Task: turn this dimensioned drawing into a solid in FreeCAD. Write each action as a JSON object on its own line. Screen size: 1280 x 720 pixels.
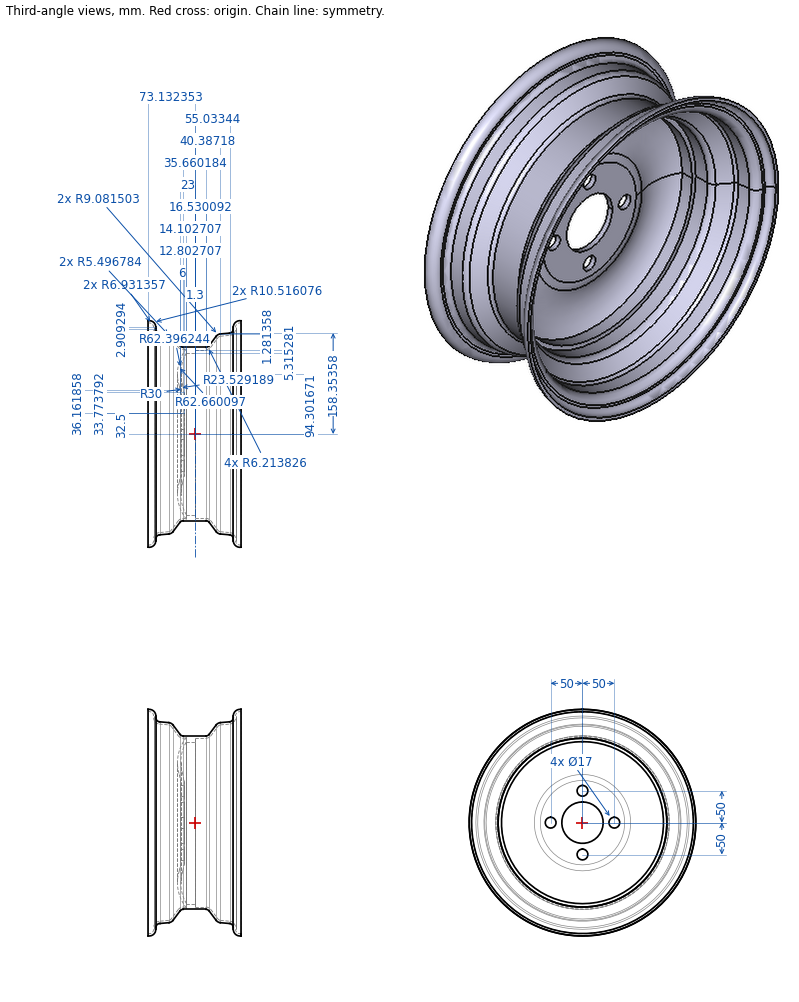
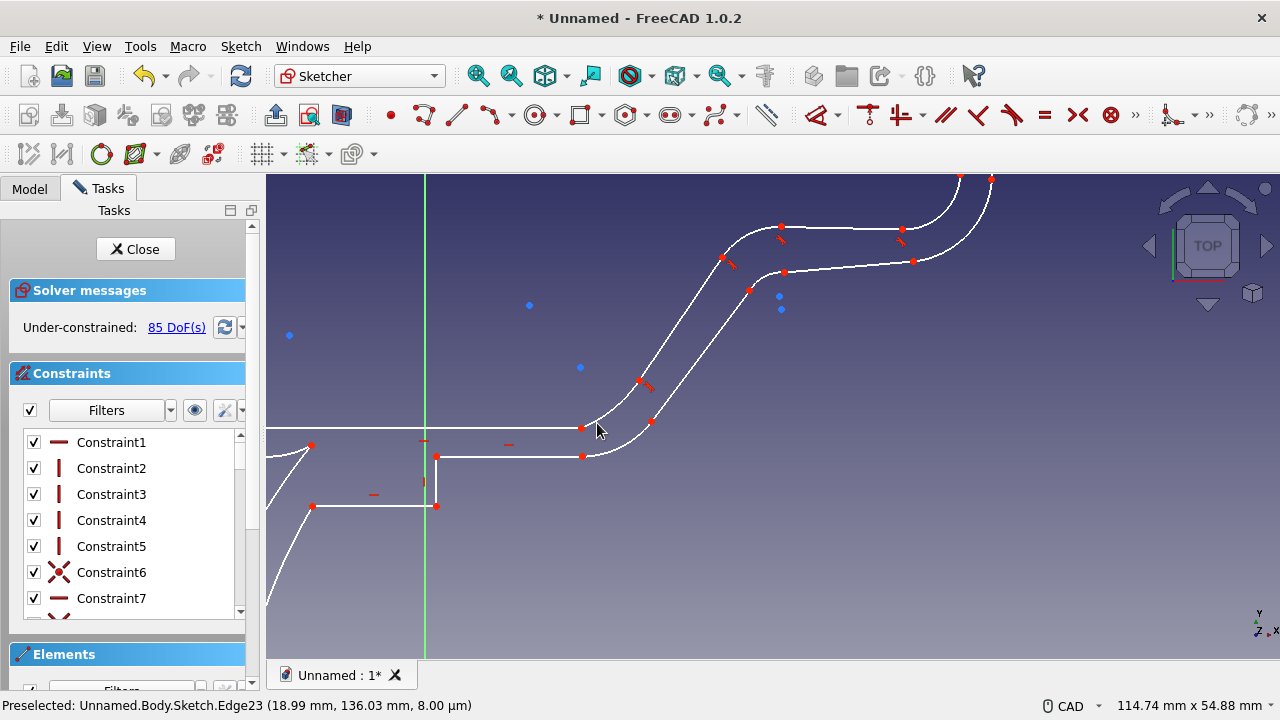
{"action": "left_click", "coordinate": [487, 428]}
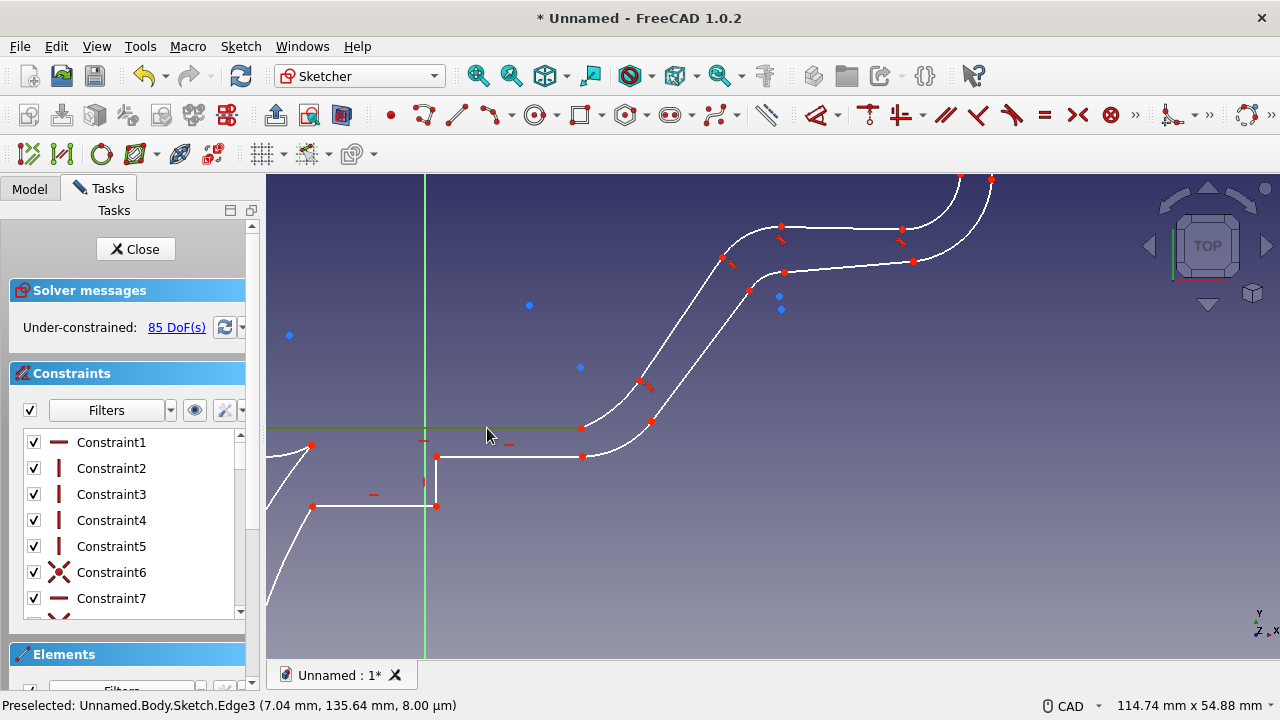
{"action": "left_click", "coordinate": [602, 417]}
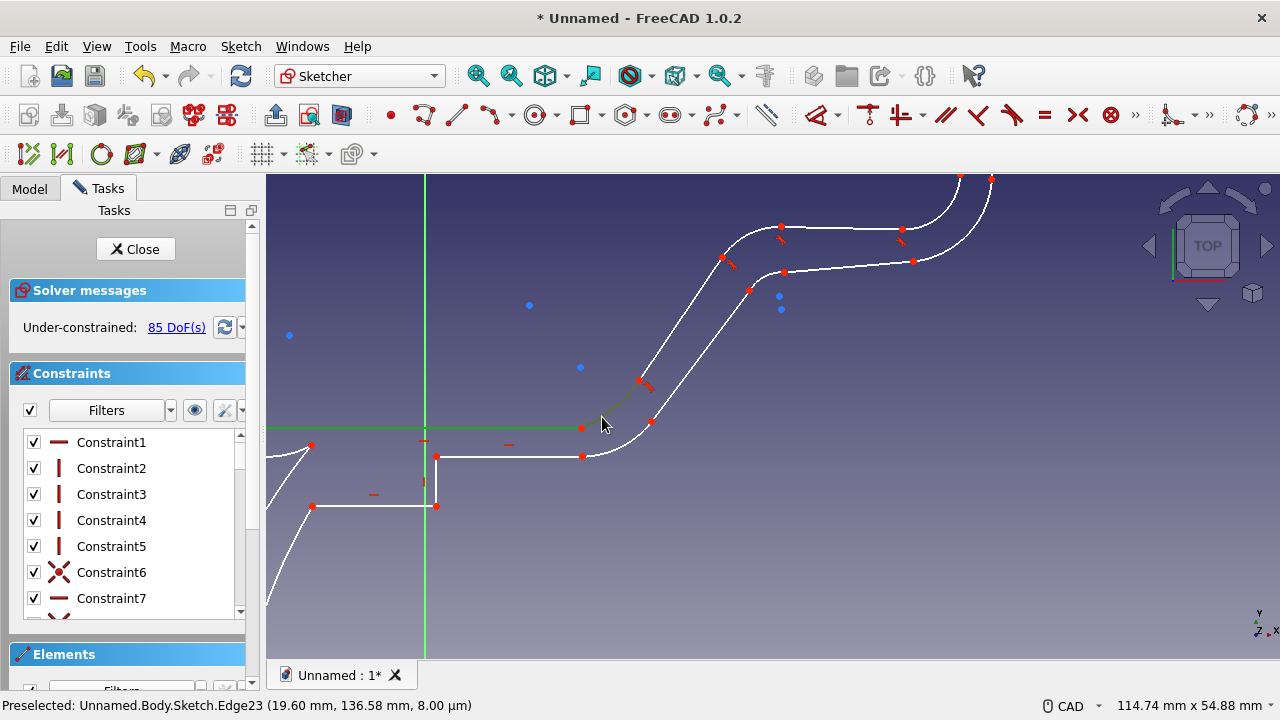
{"action": "key", "text": "t"}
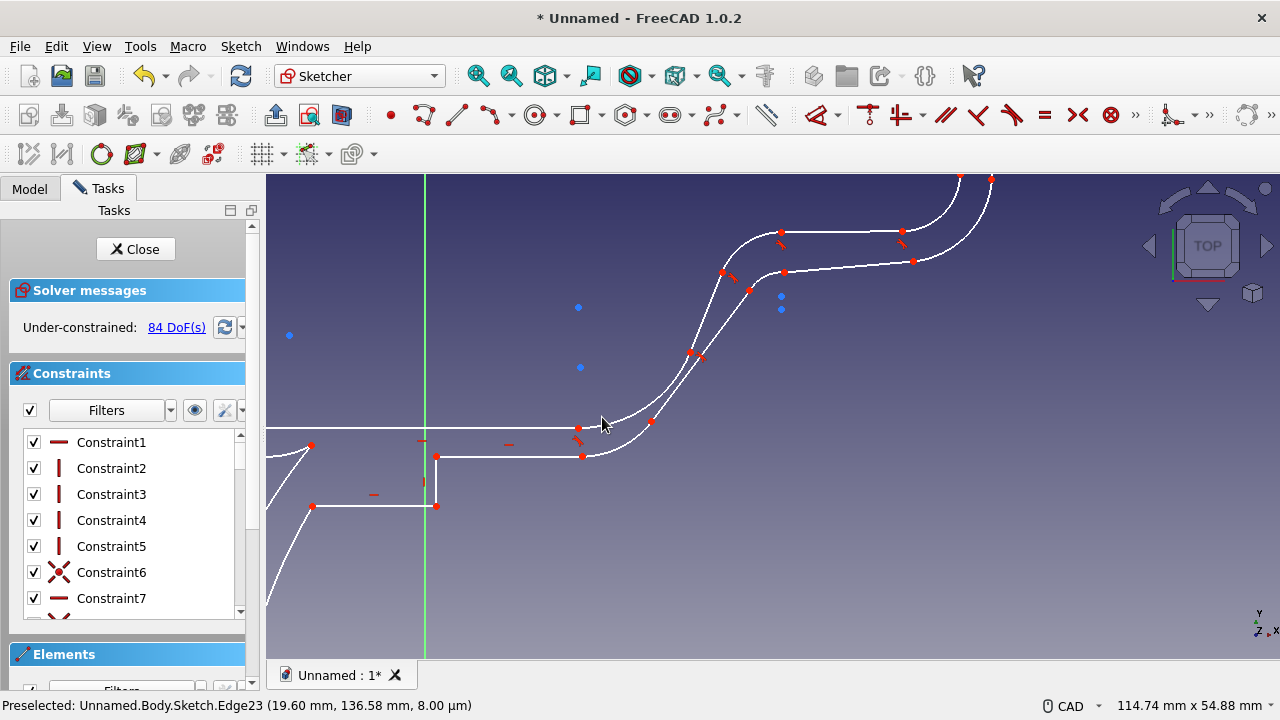
{"action": "left_click", "coordinate": [485, 428]}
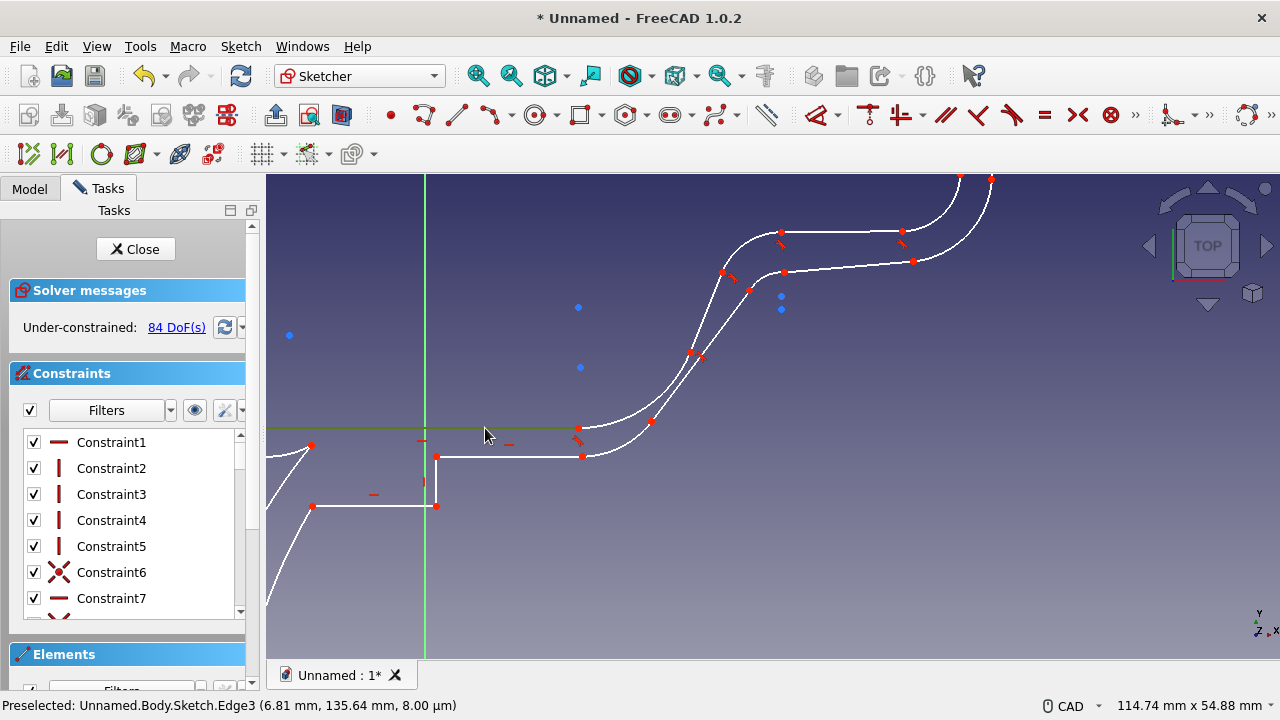
{"action": "scroll", "coordinate": [775, 309], "scroll_direction": "down", "scroll_amount": 8}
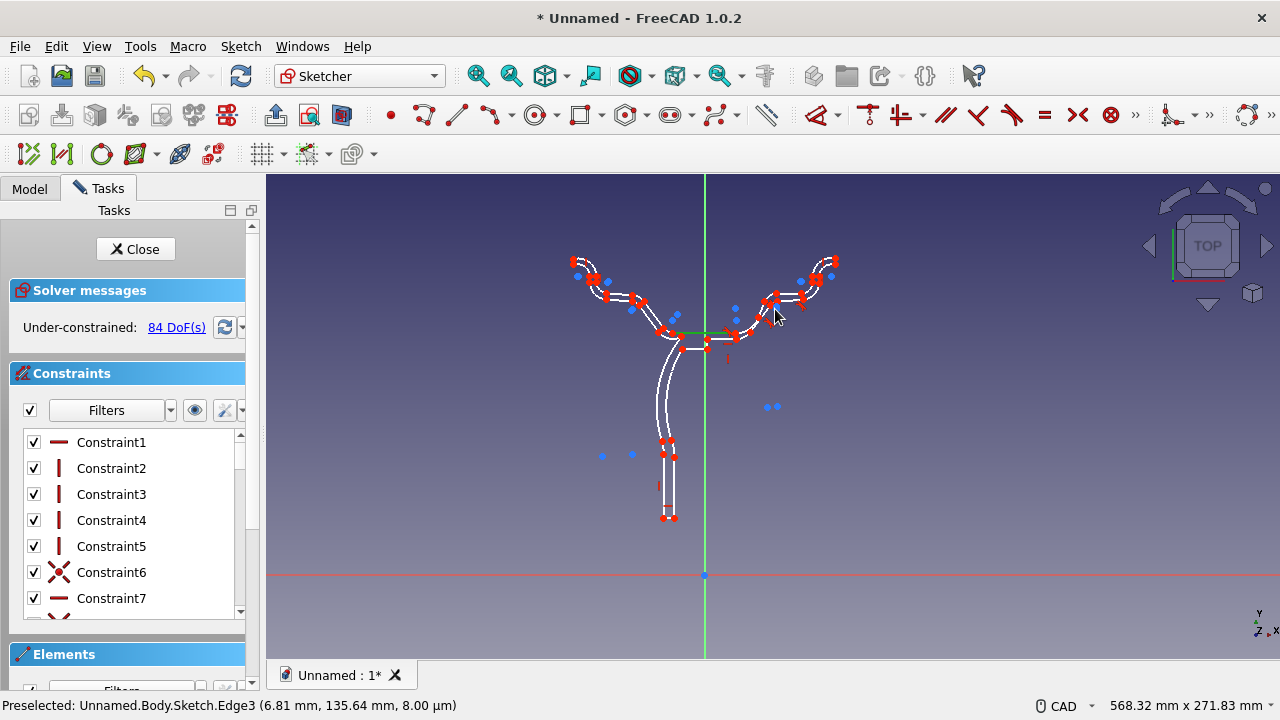
{"action": "scroll", "coordinate": [666, 330], "scroll_direction": "up", "scroll_amount": 8}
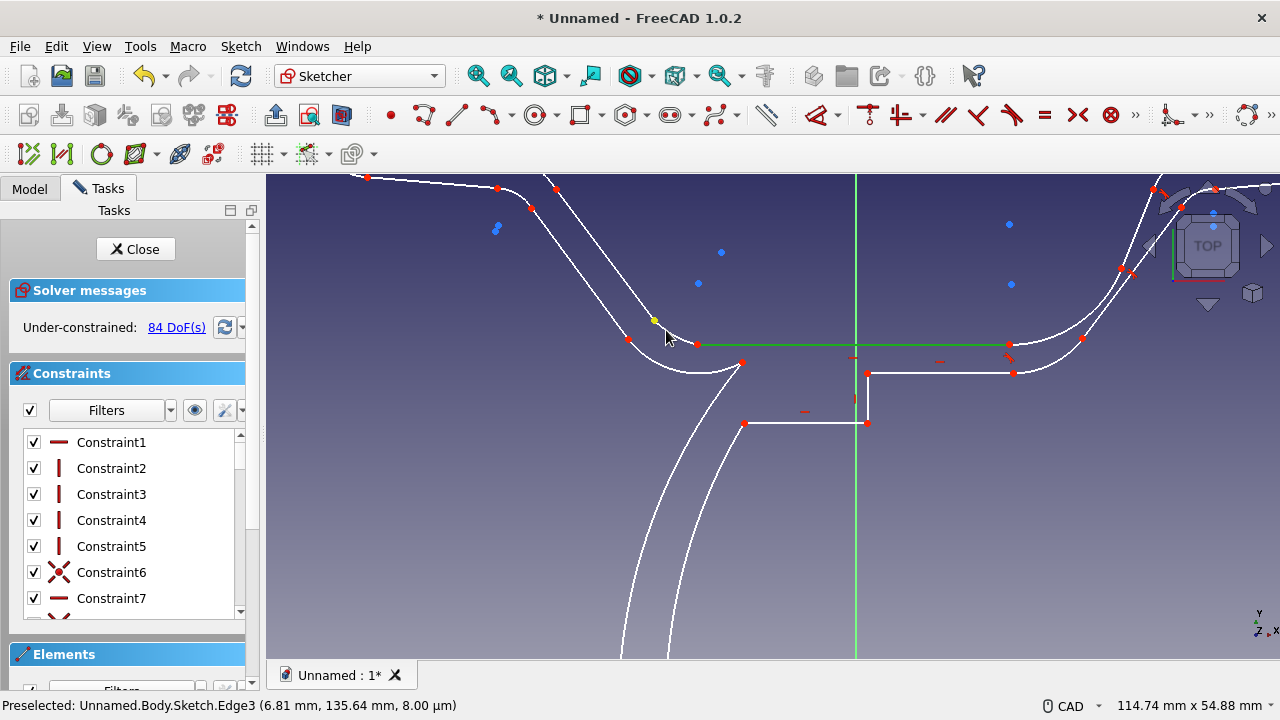
{"action": "left_click", "coordinate": [666, 330]}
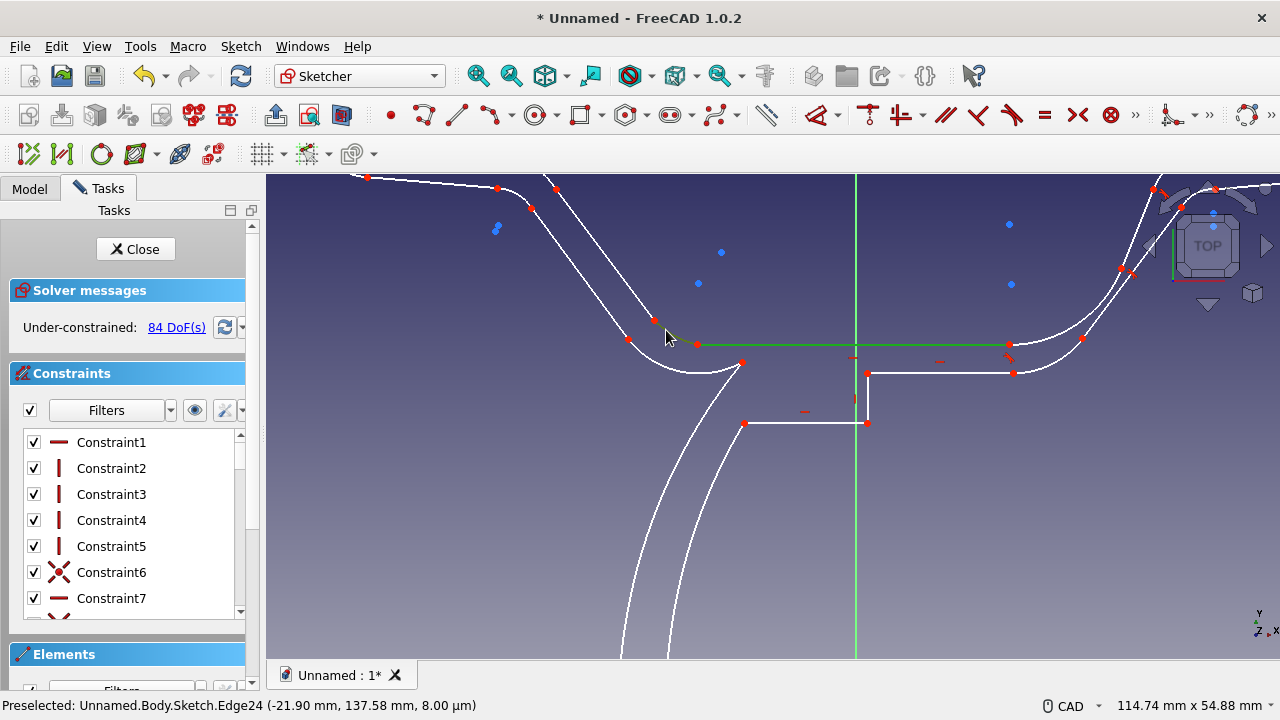
{"action": "key", "text": "t"}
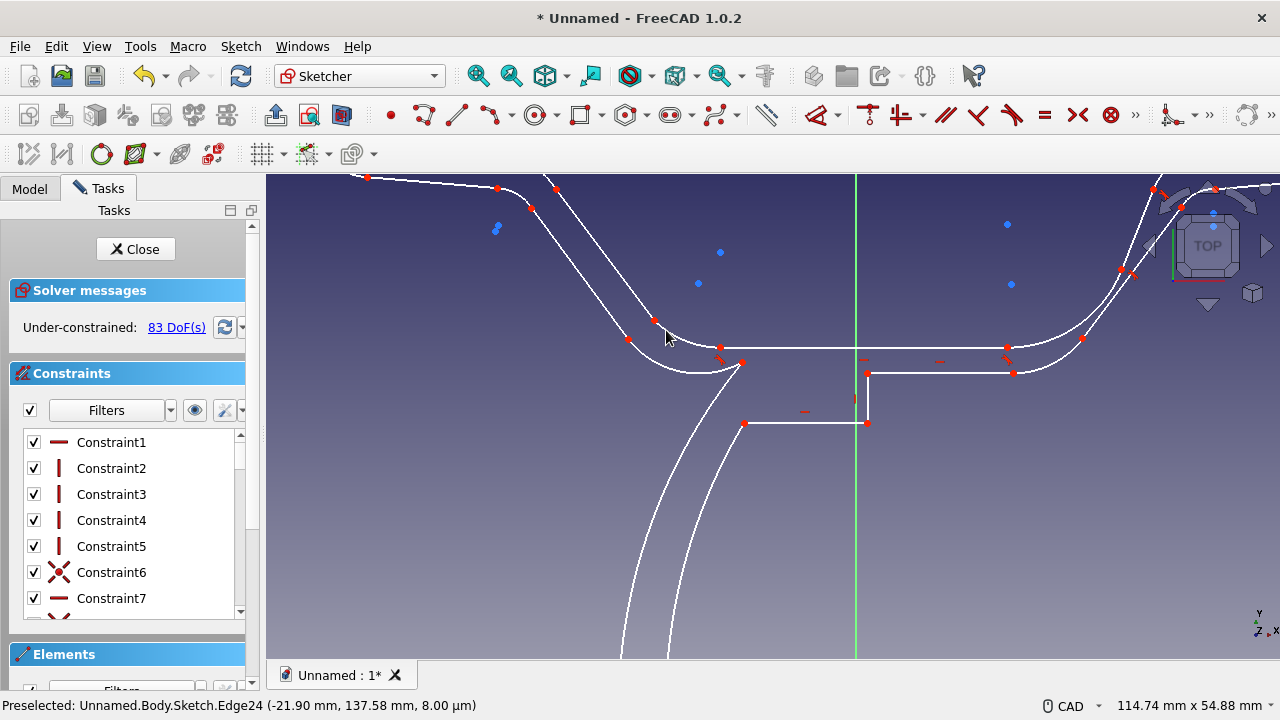
{"action": "left_click", "coordinate": [625, 281]}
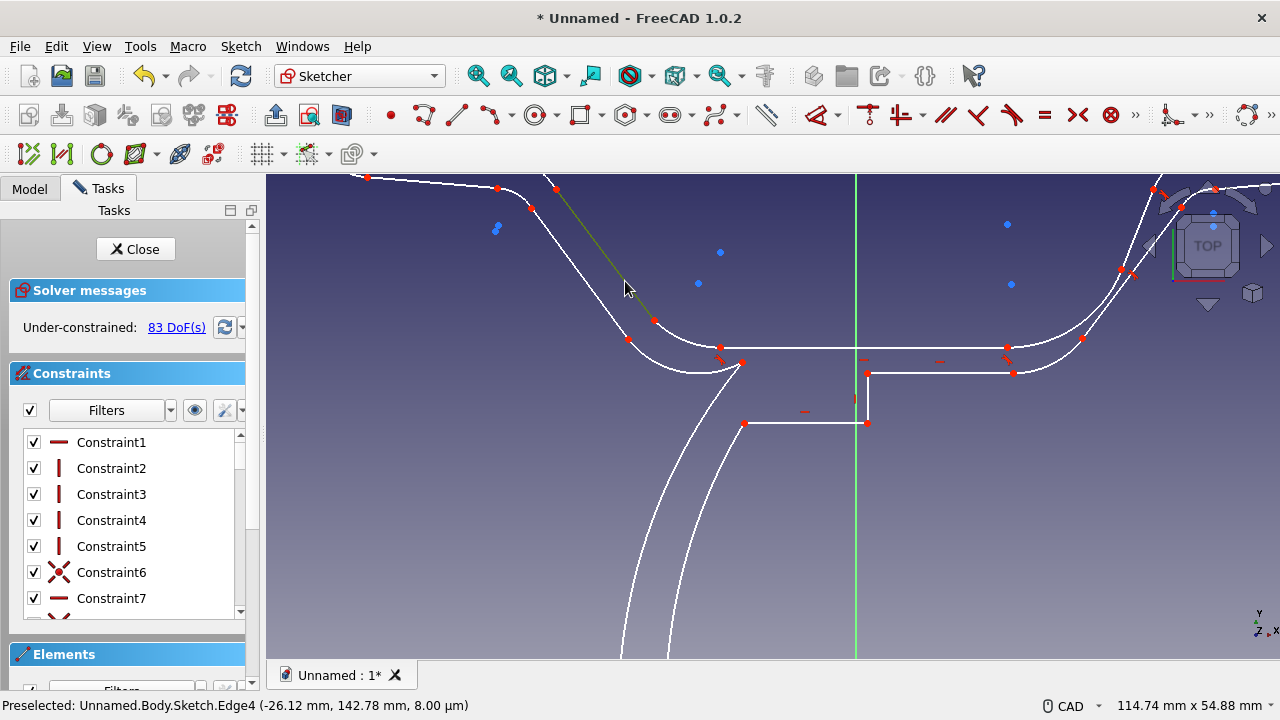
{"action": "left_click", "coordinate": [672, 334]}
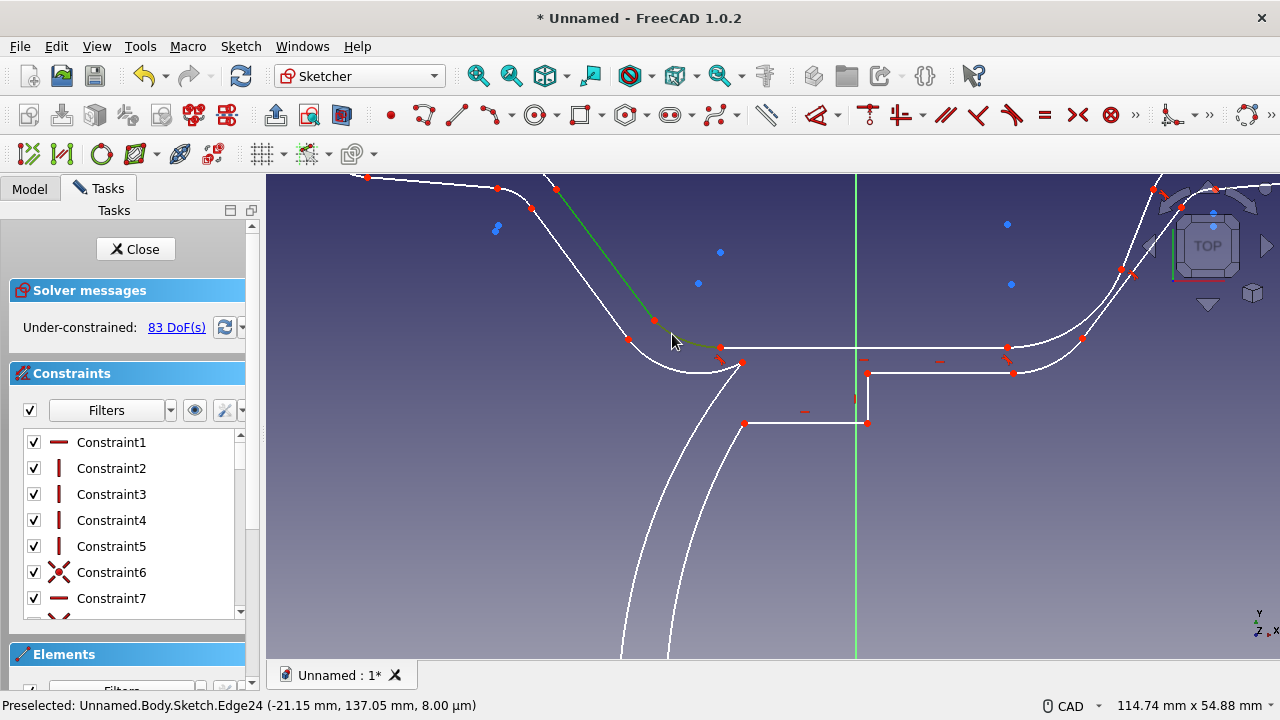
{"action": "key", "text": "t"}